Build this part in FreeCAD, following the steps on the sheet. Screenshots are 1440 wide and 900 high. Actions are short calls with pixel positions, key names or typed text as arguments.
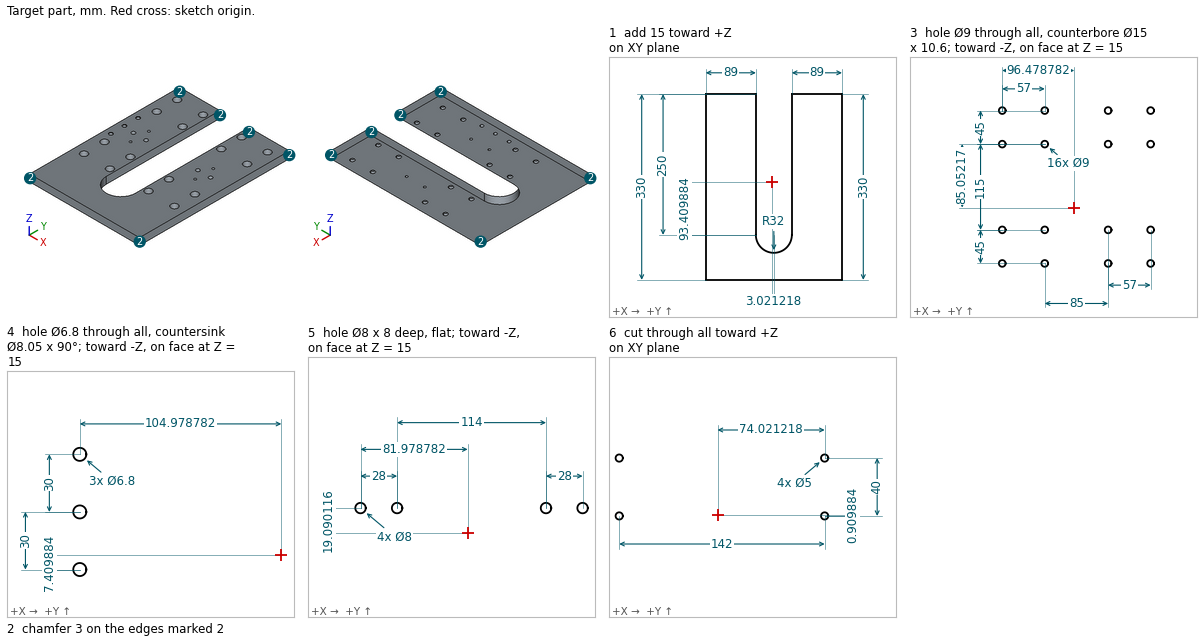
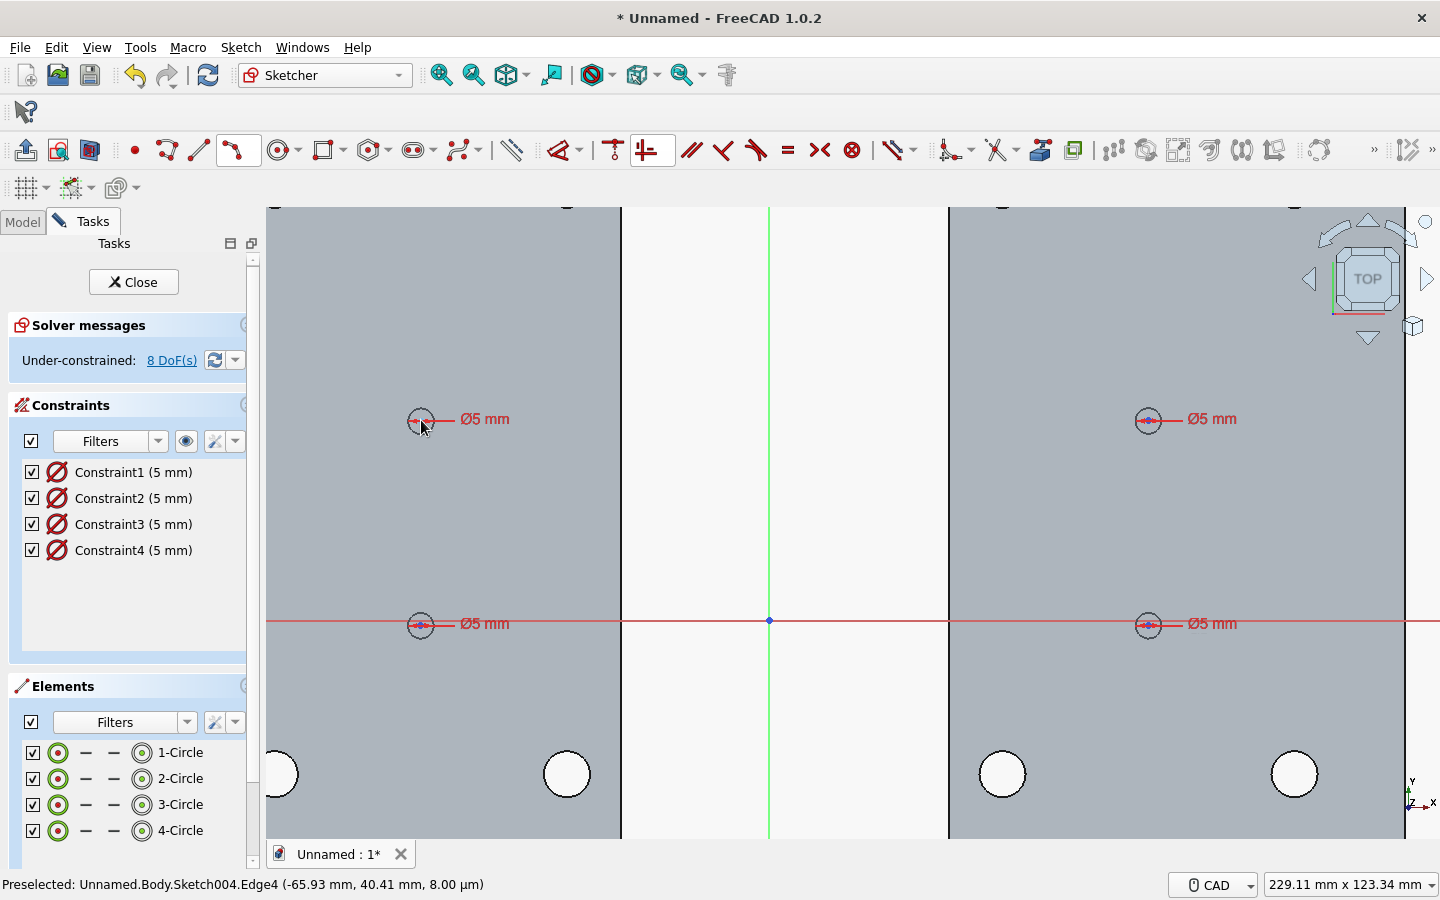
click(1148, 421)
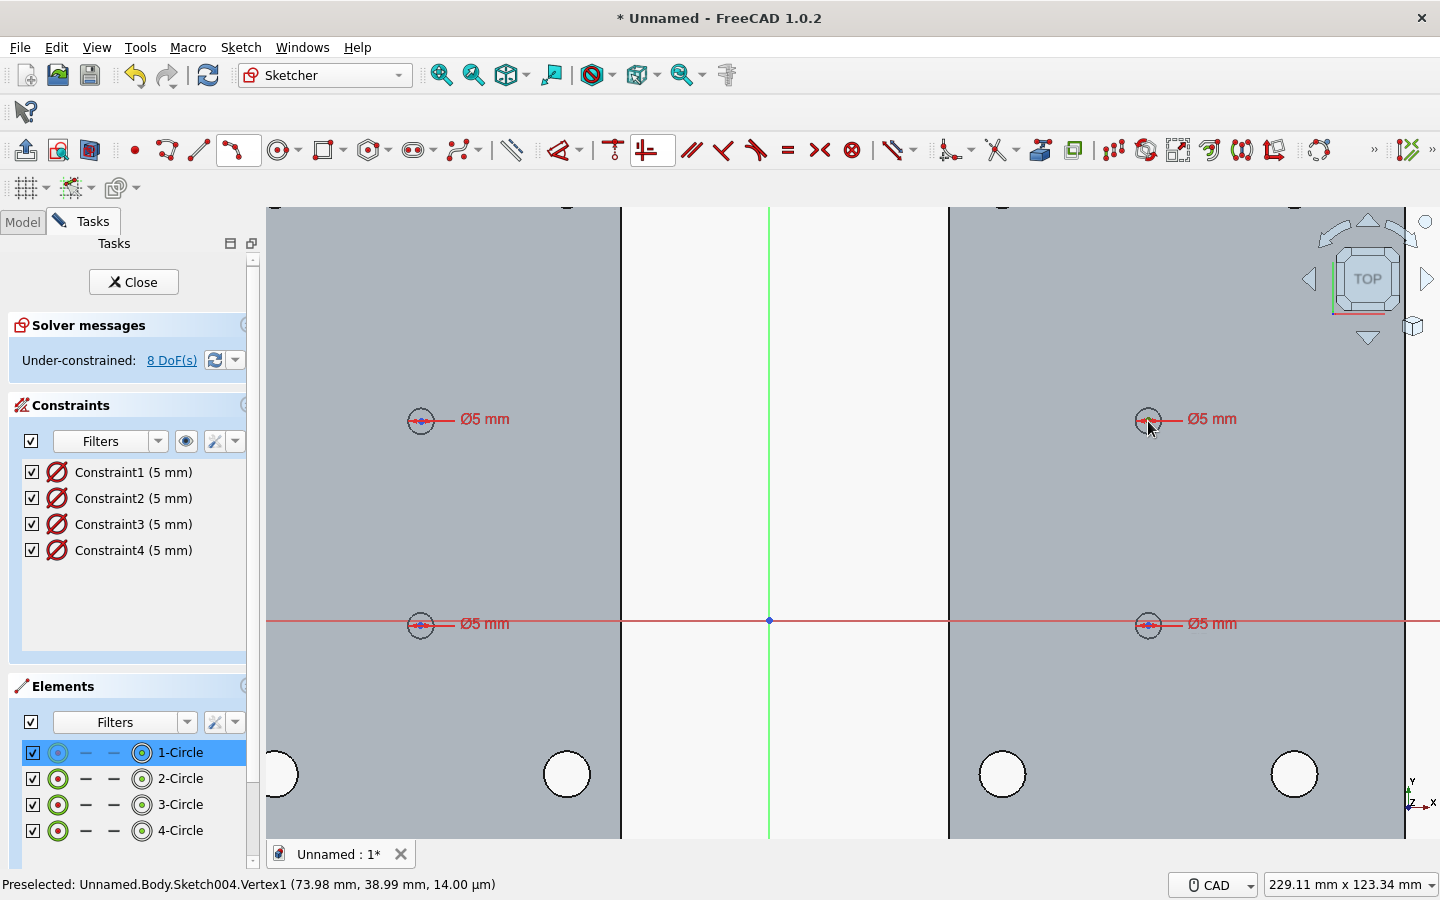
click(1149, 626)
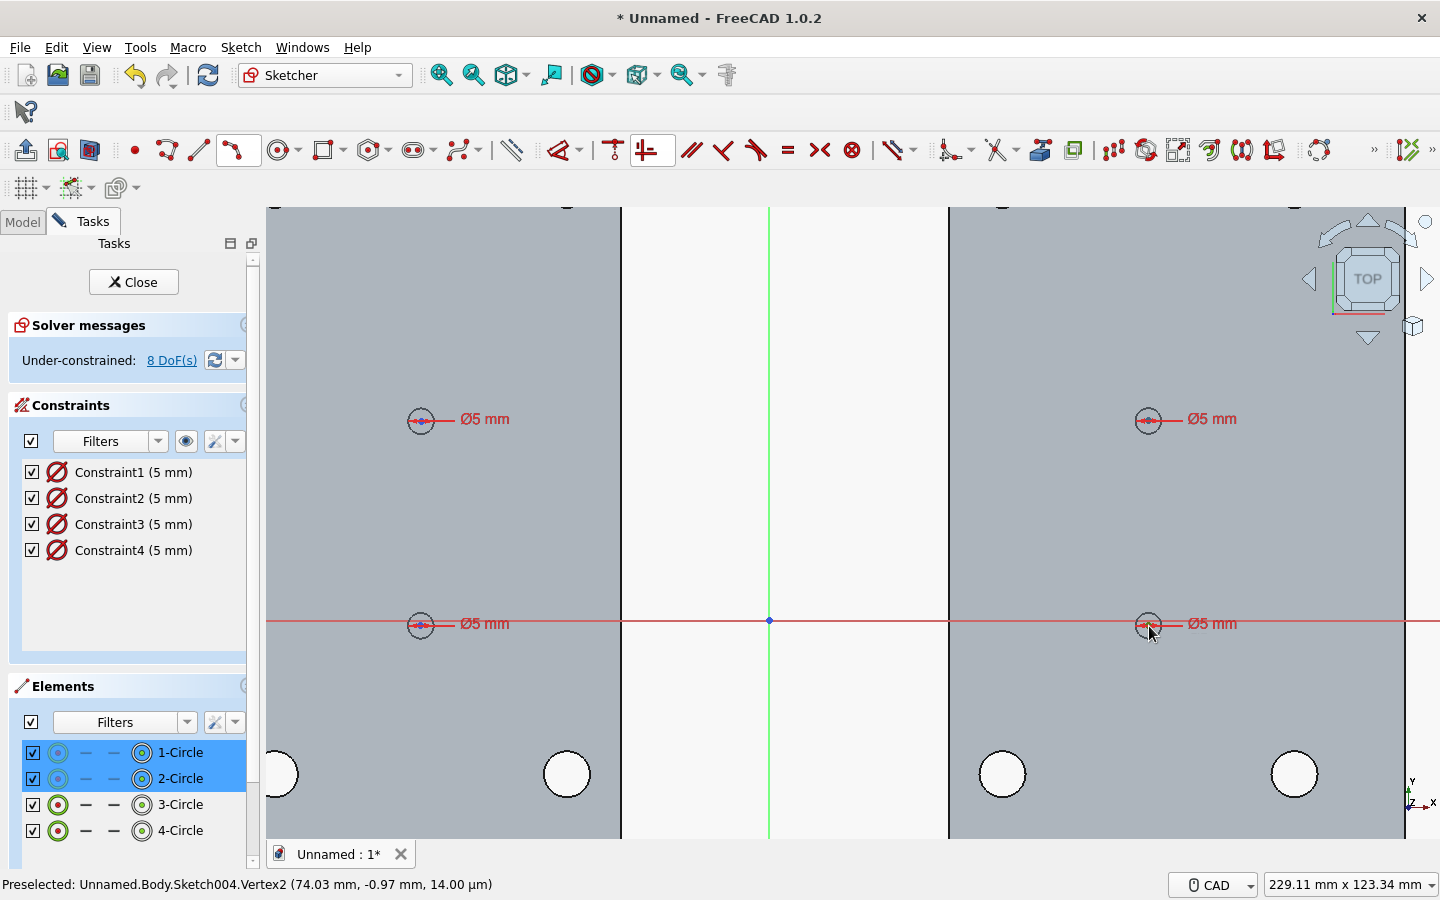
key(v)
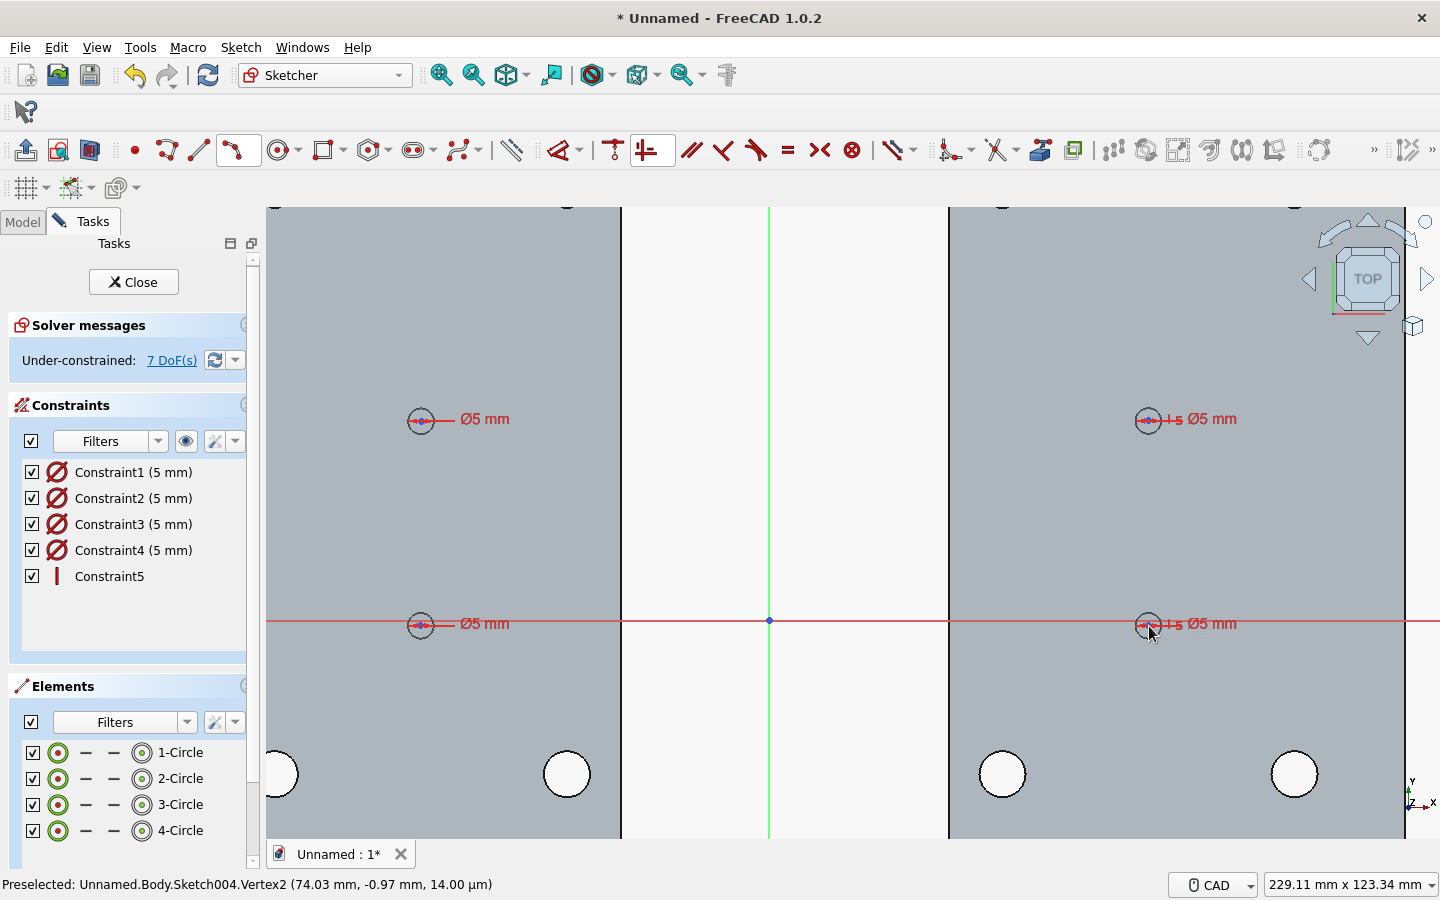
click(1148, 626)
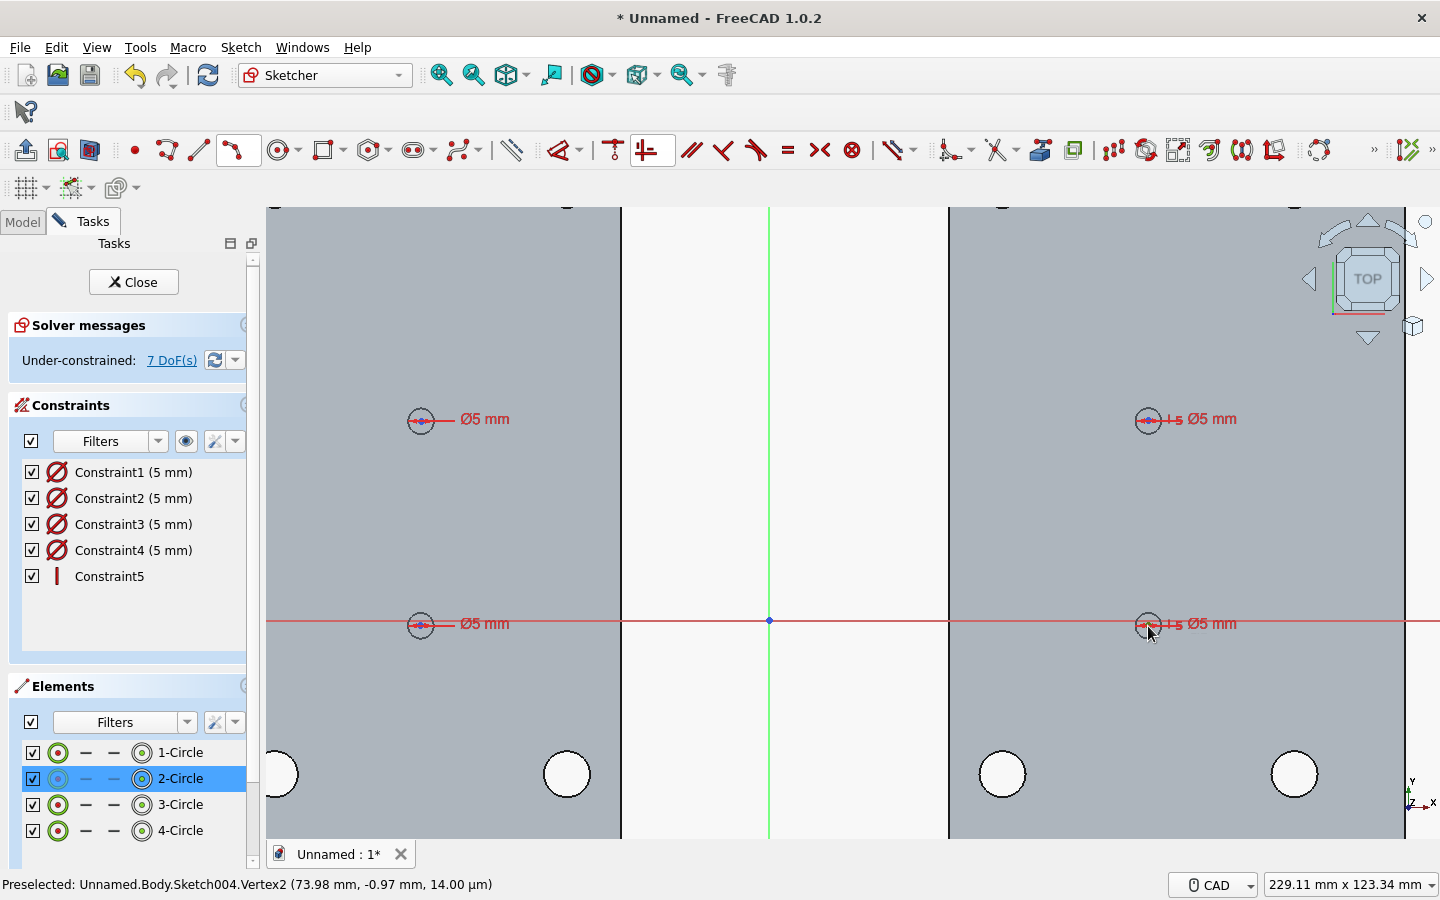
click(421, 626)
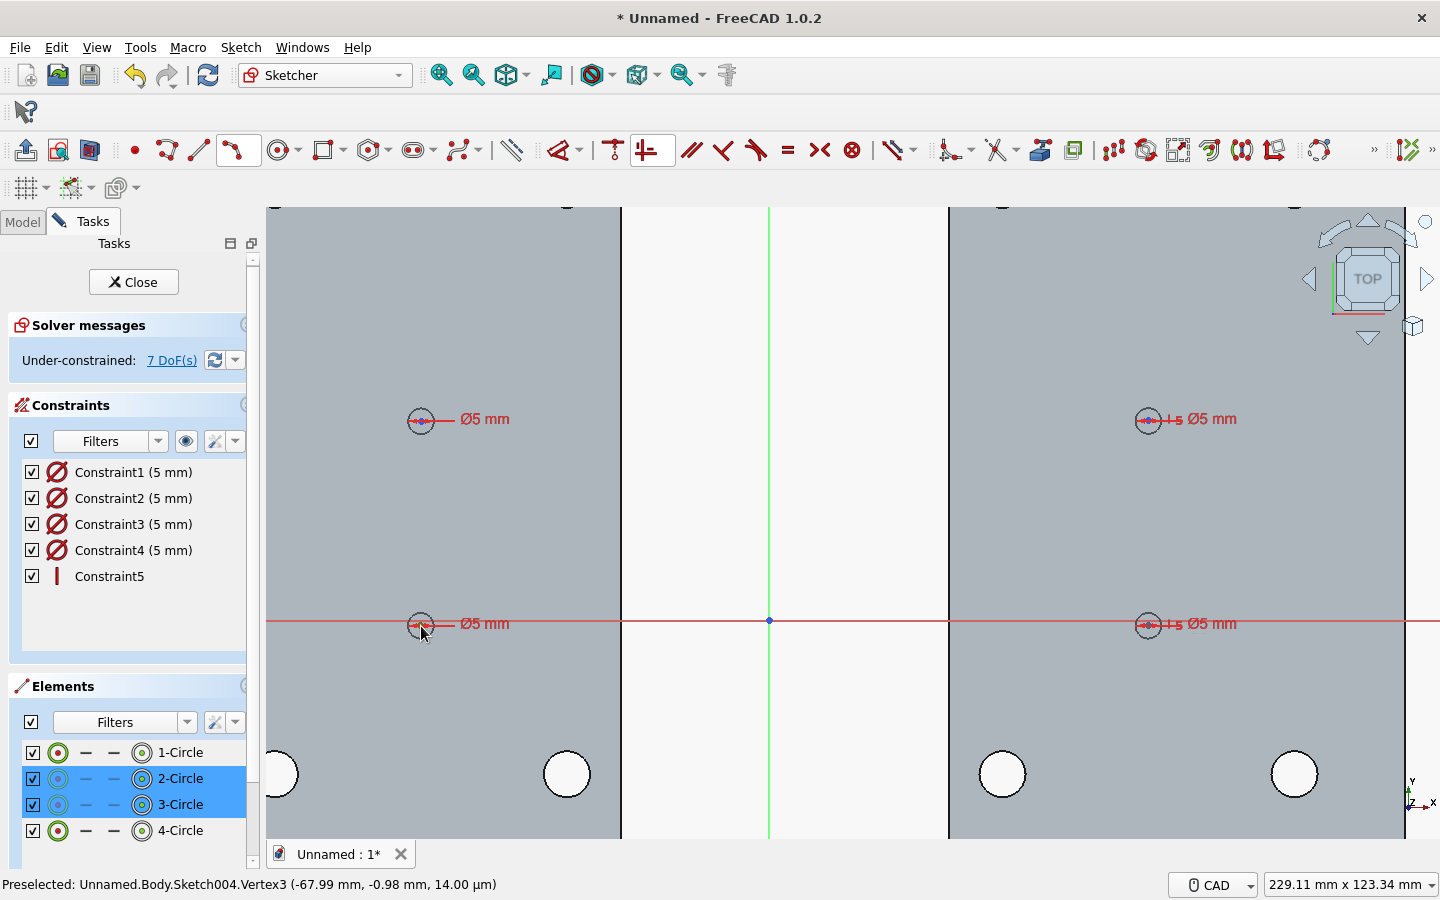
key(h)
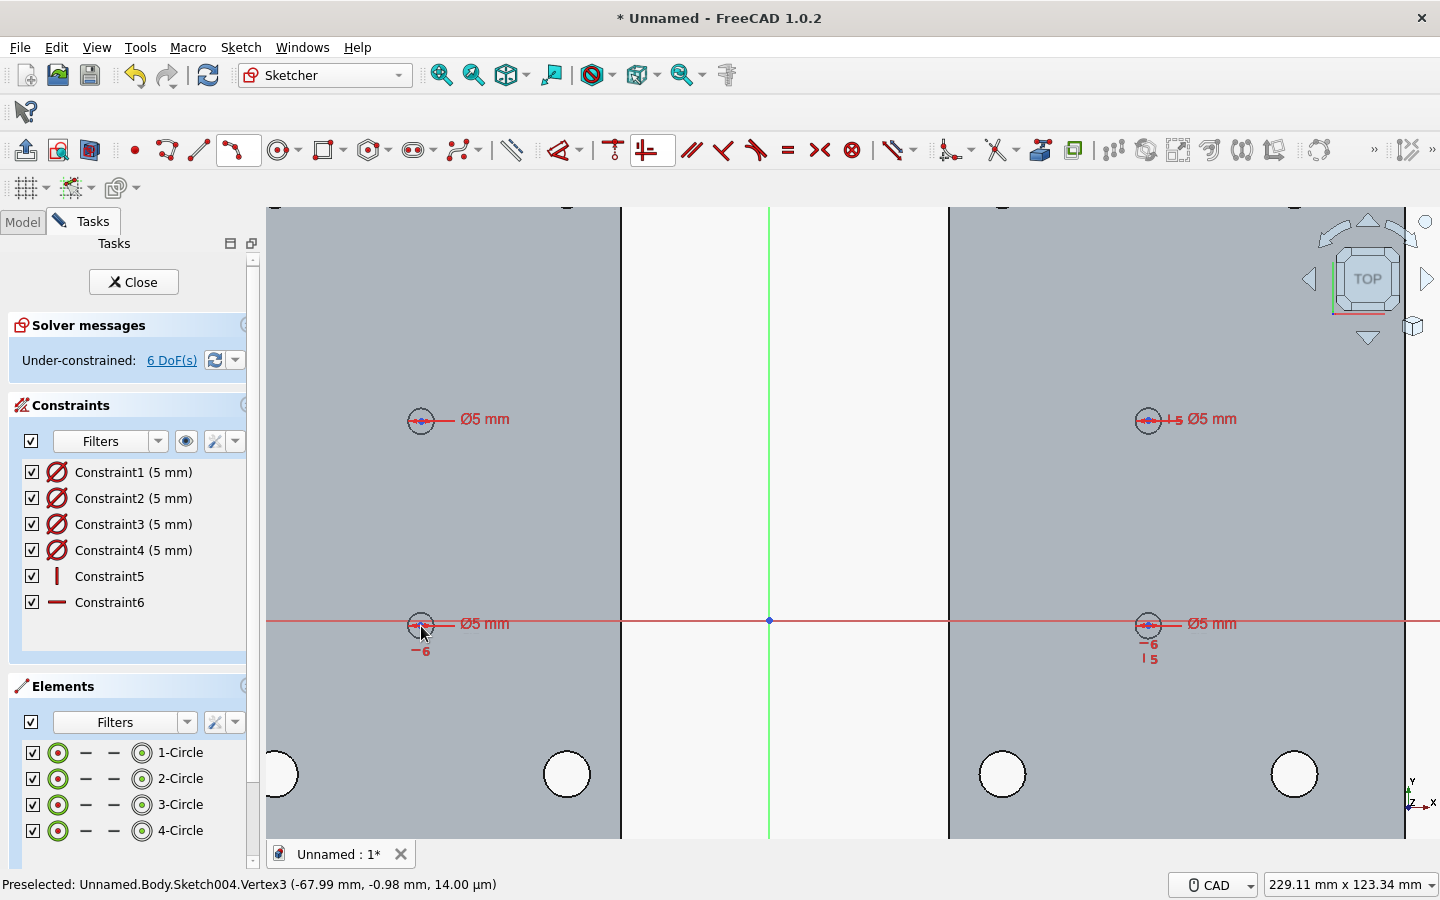
click(421, 626)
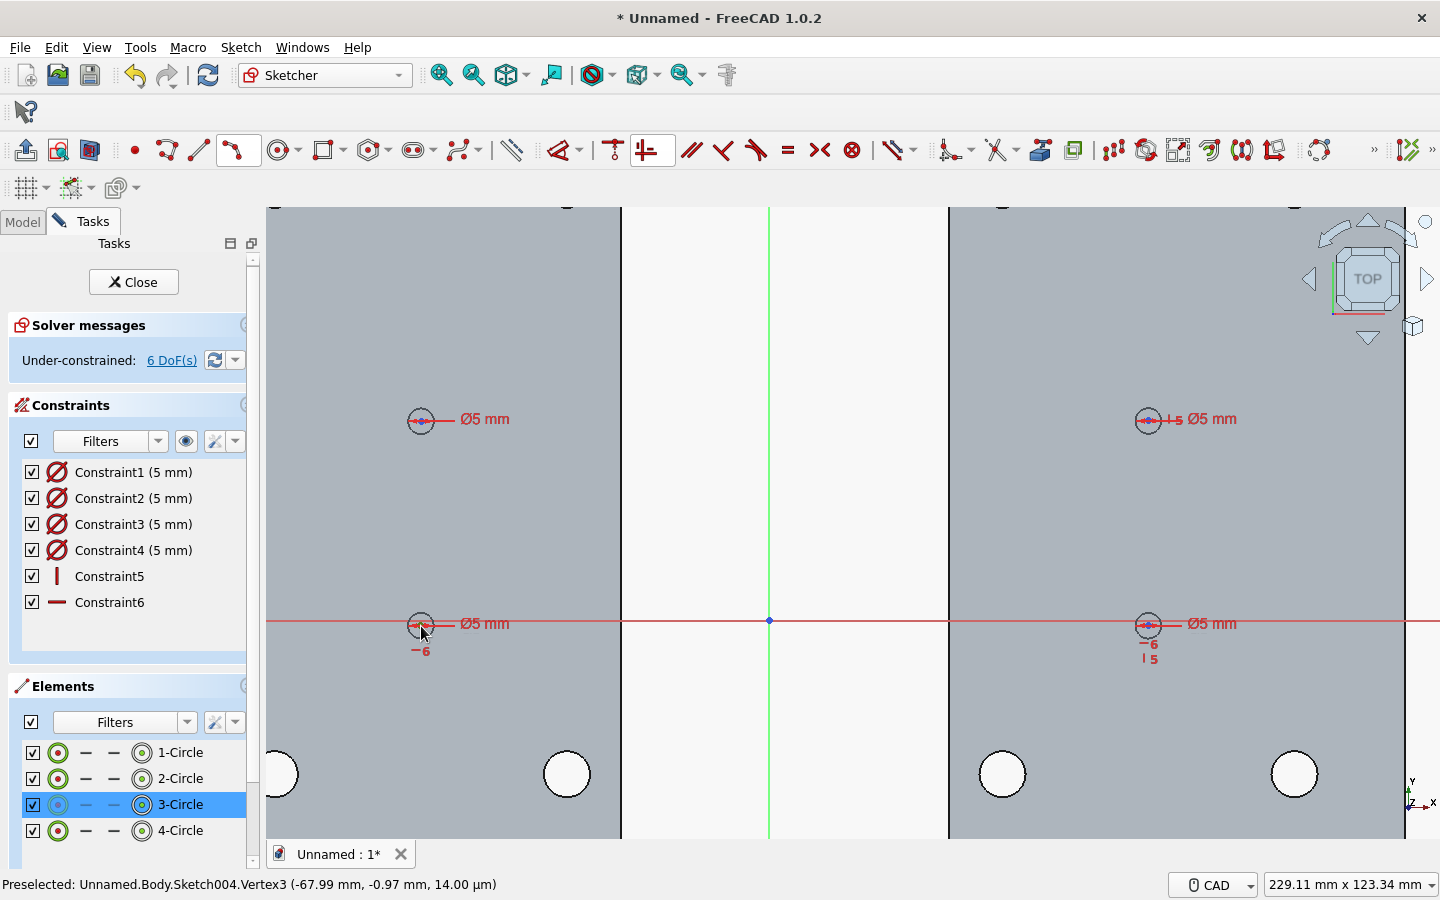
click(421, 421)